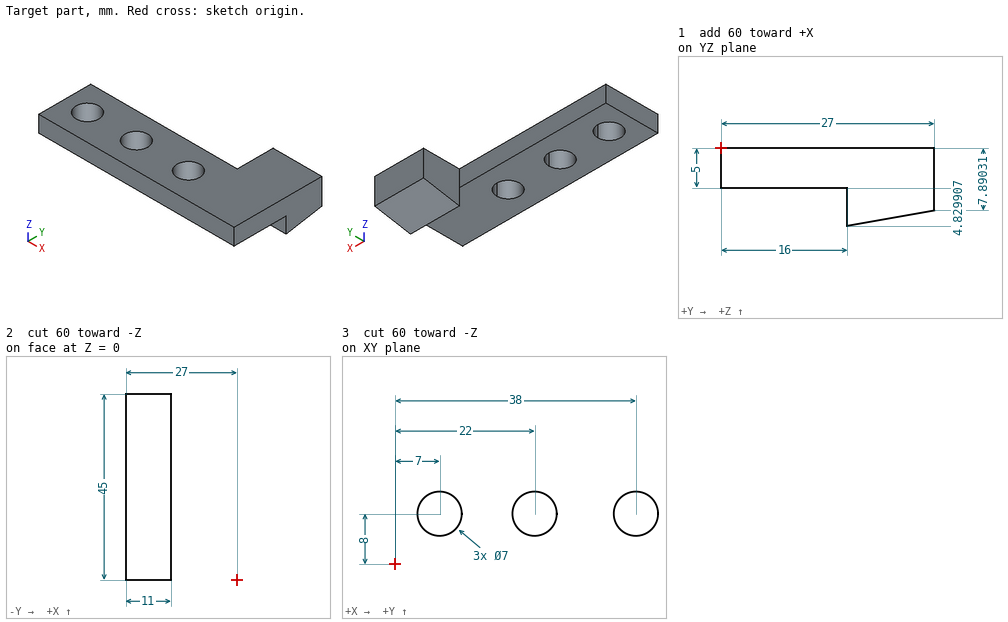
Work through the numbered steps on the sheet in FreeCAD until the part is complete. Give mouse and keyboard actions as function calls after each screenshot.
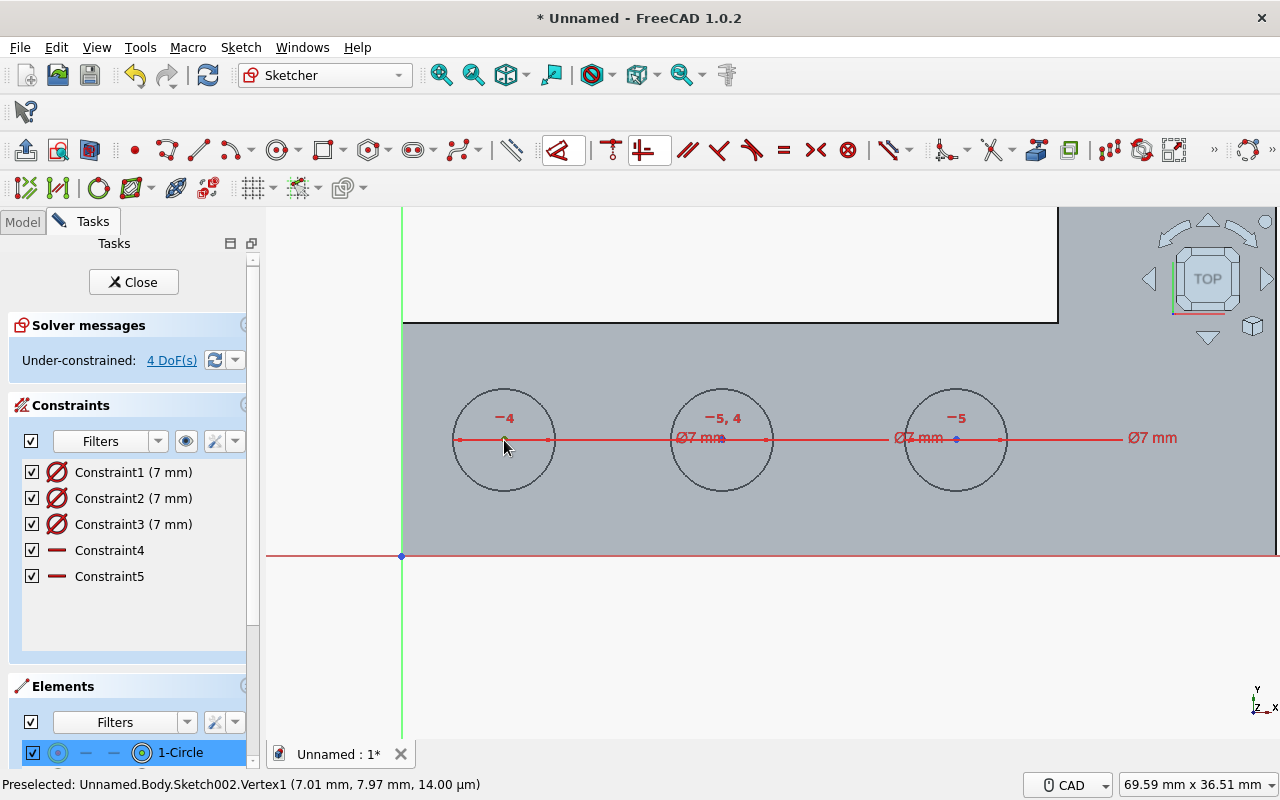
click(580, 150)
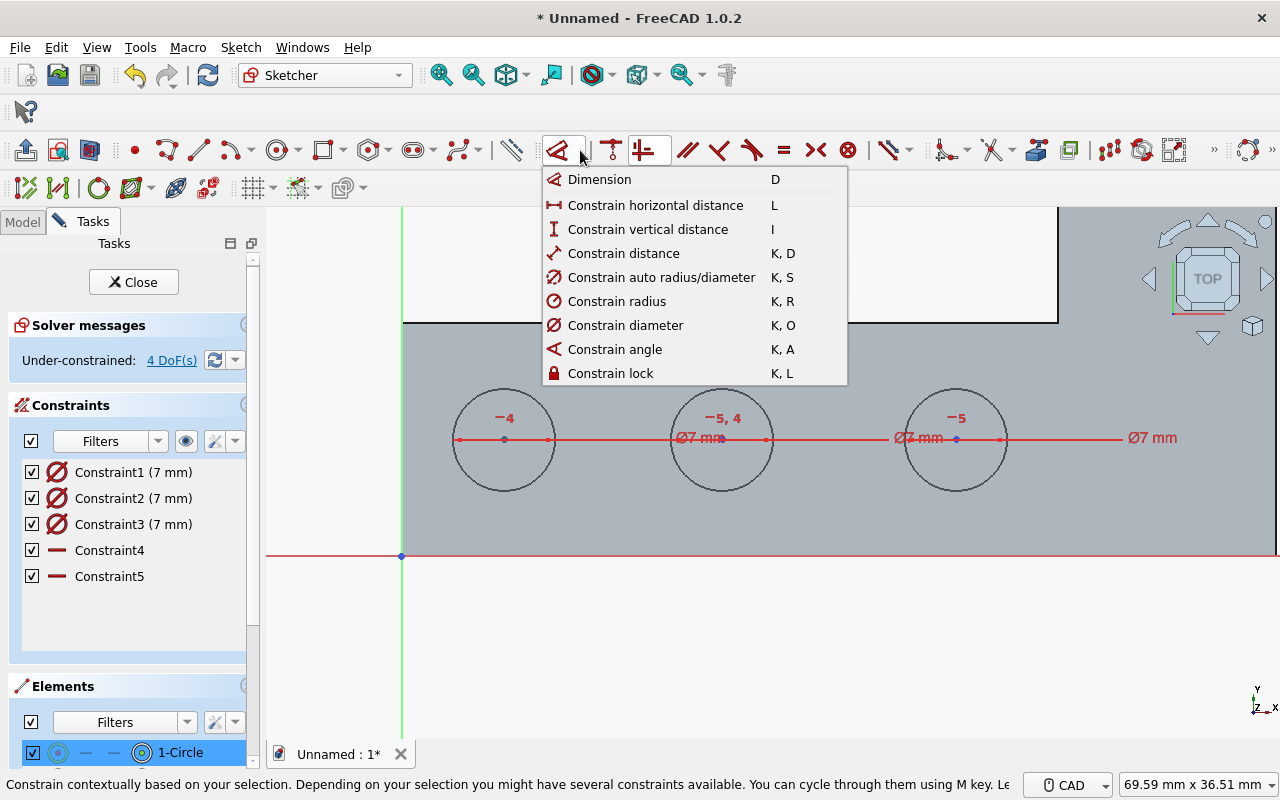
click(695, 205)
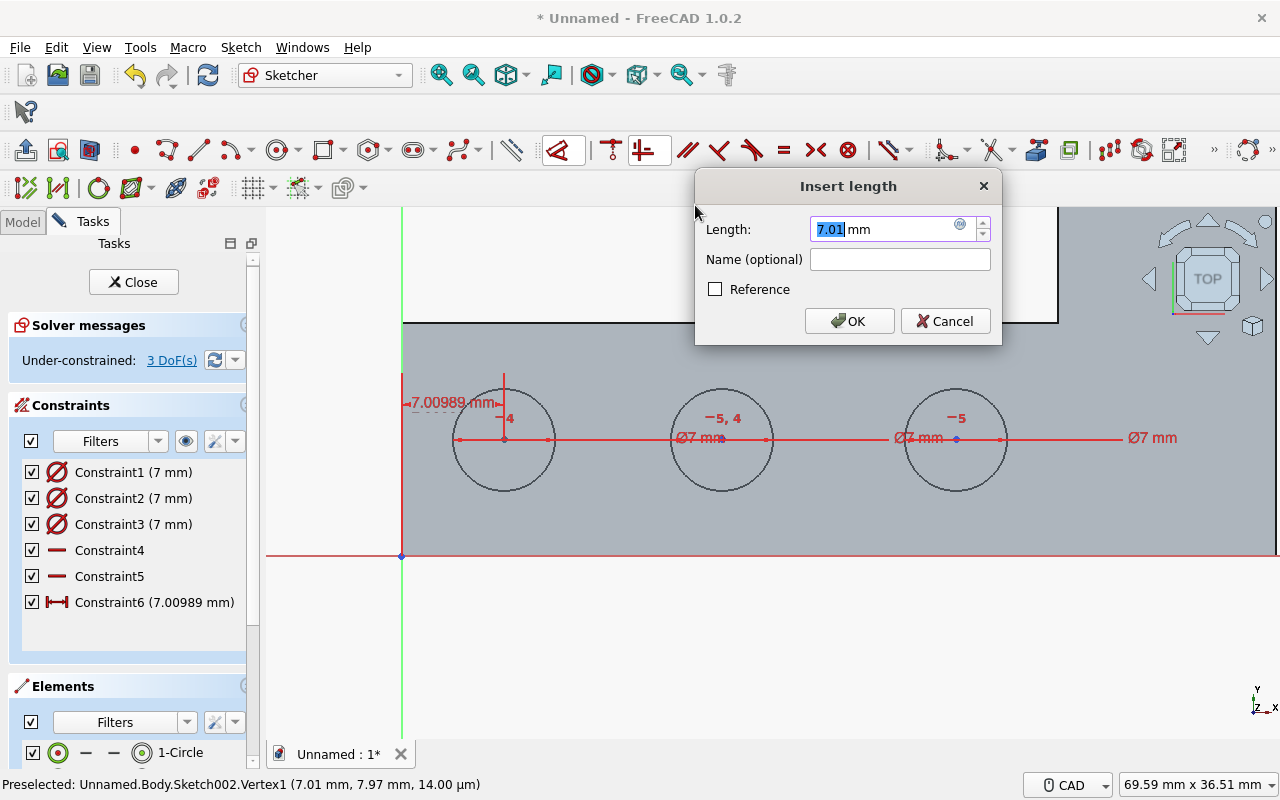
text(7)
key(Return)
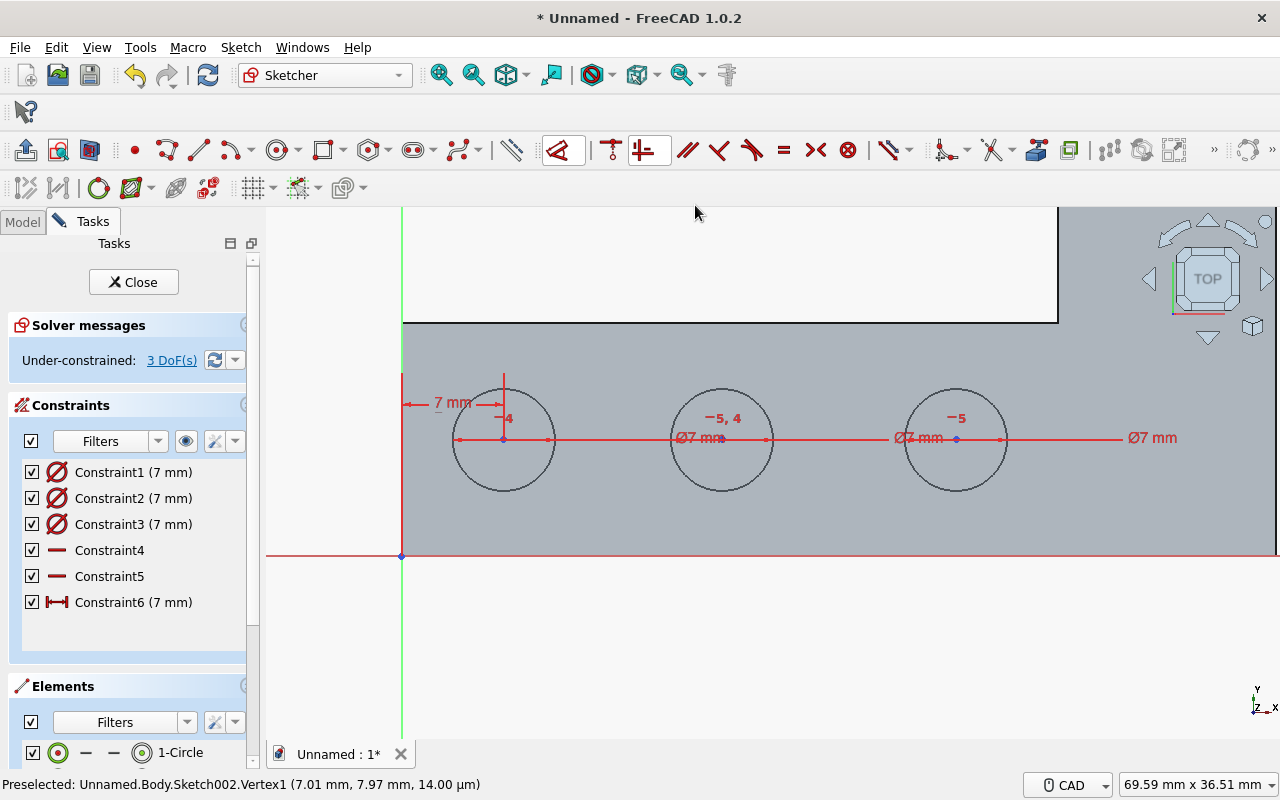
click(504, 440)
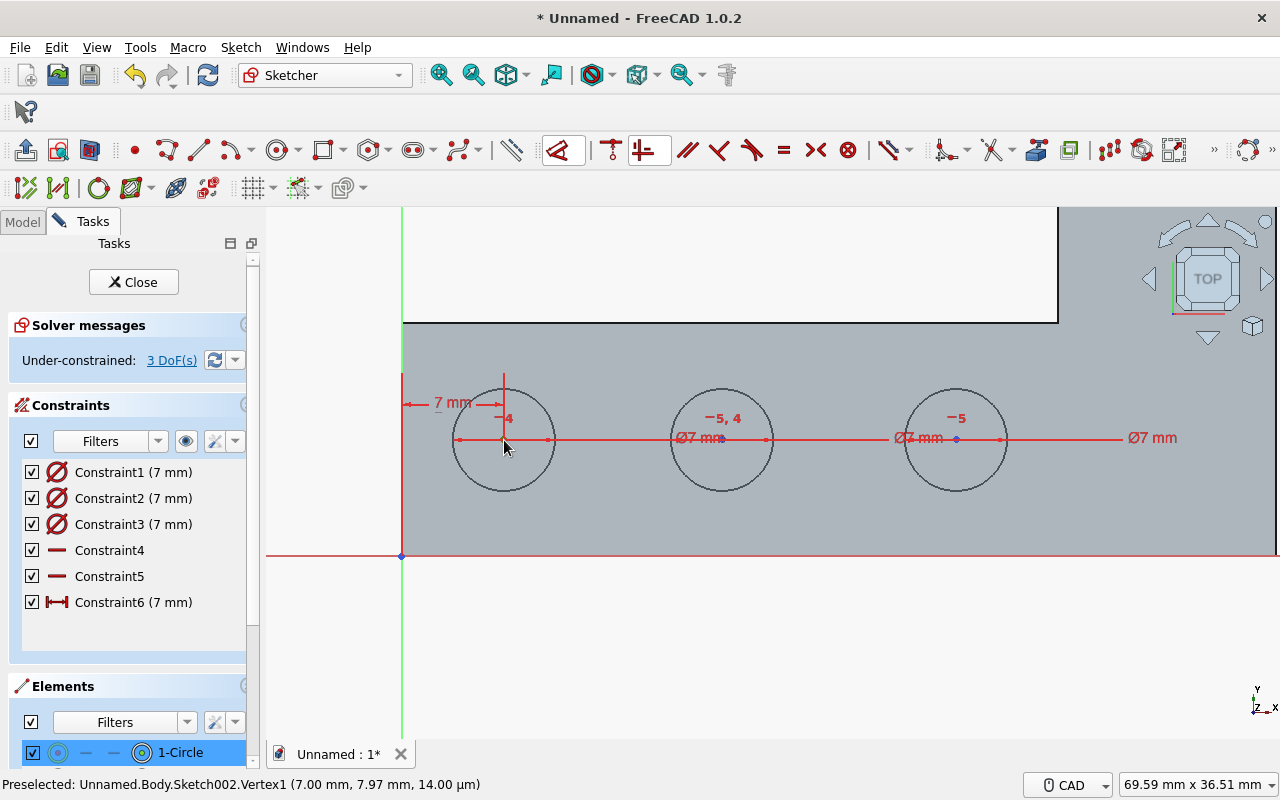
key(i)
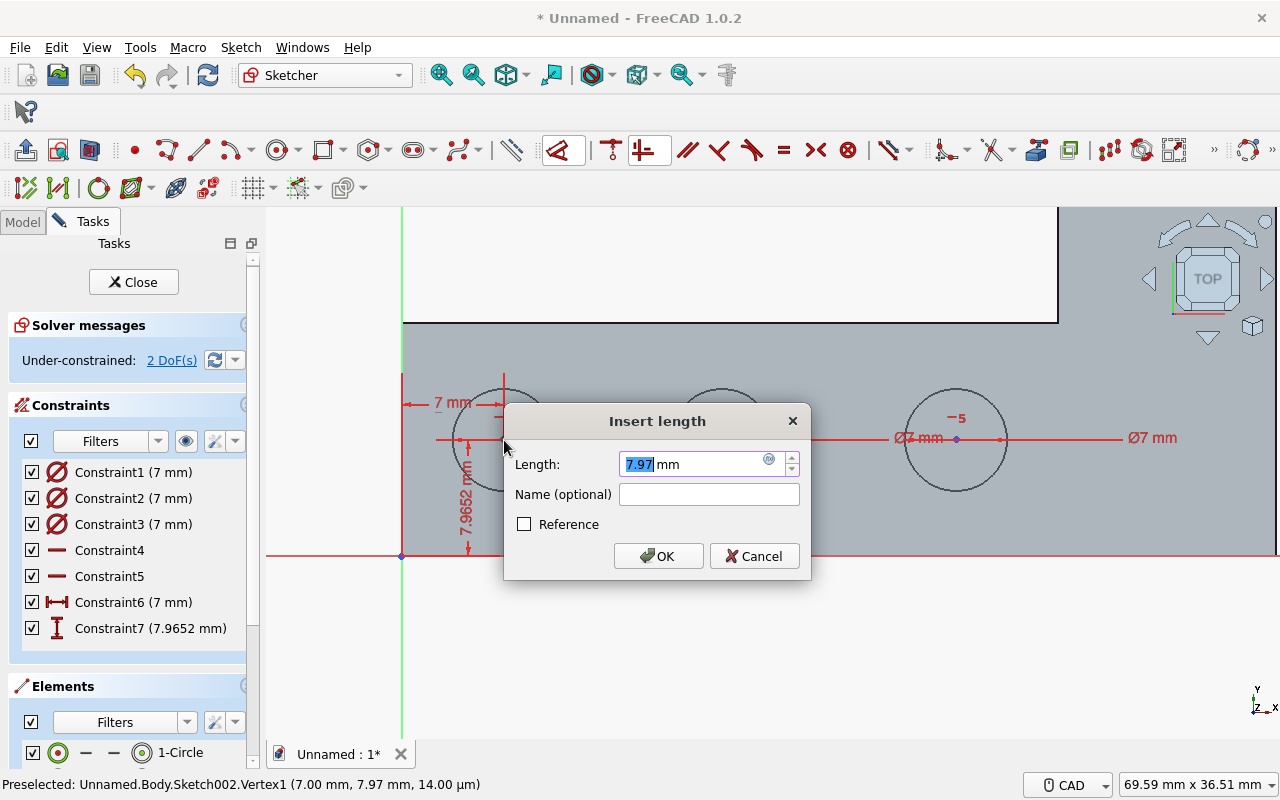
text(8)
key(Return)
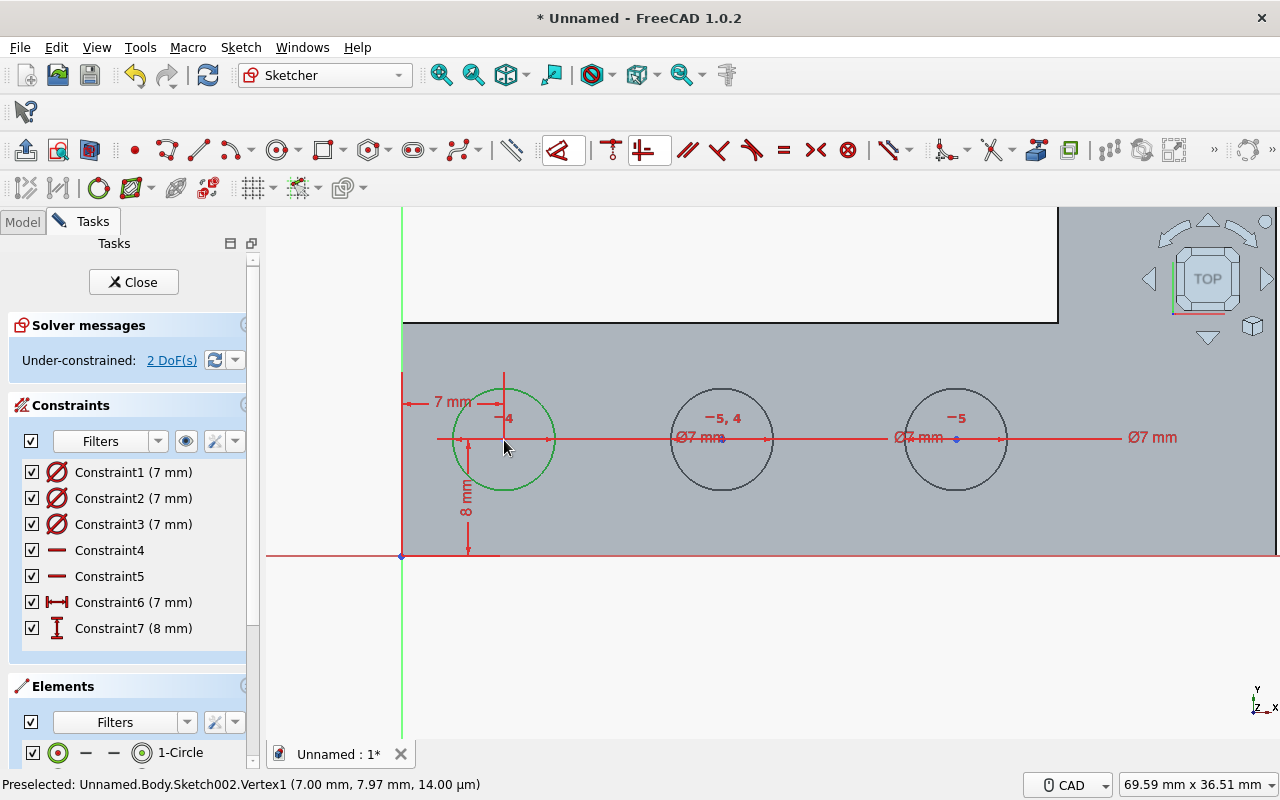
click(722, 439)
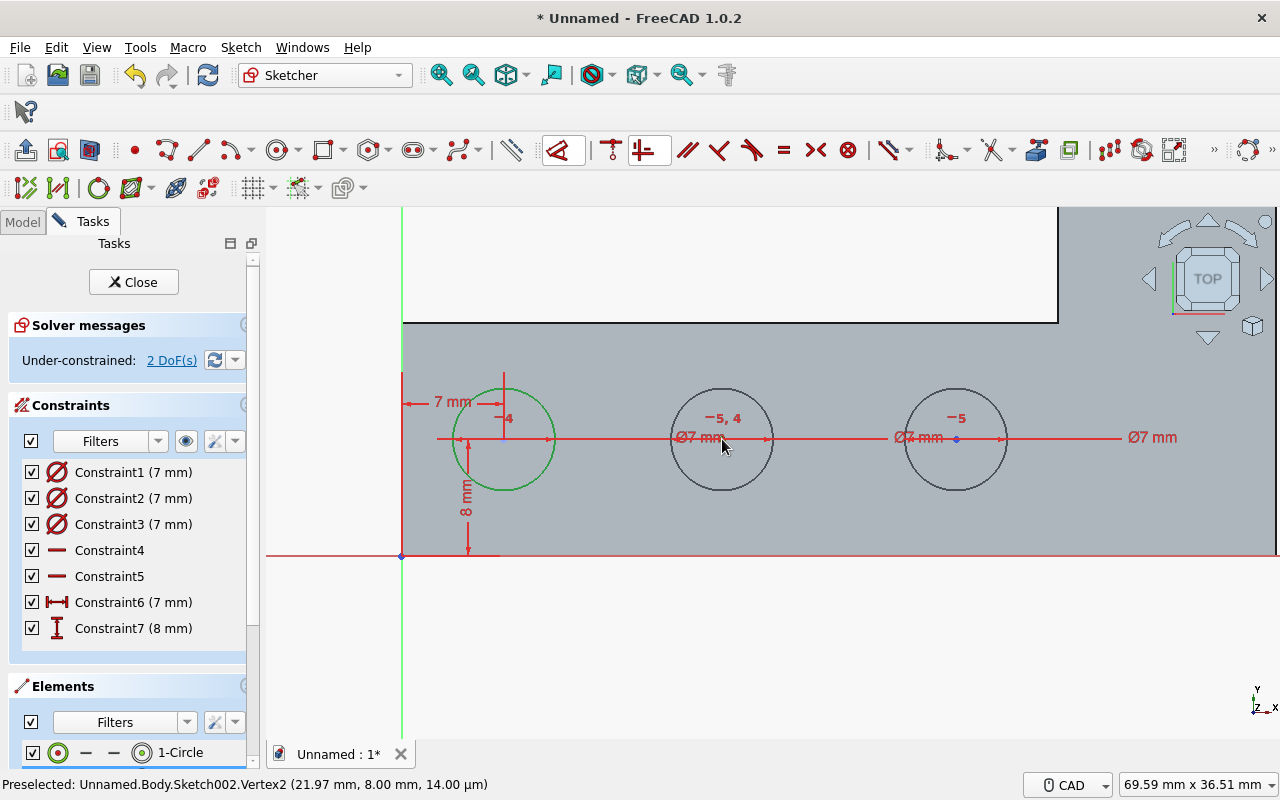
click(580, 150)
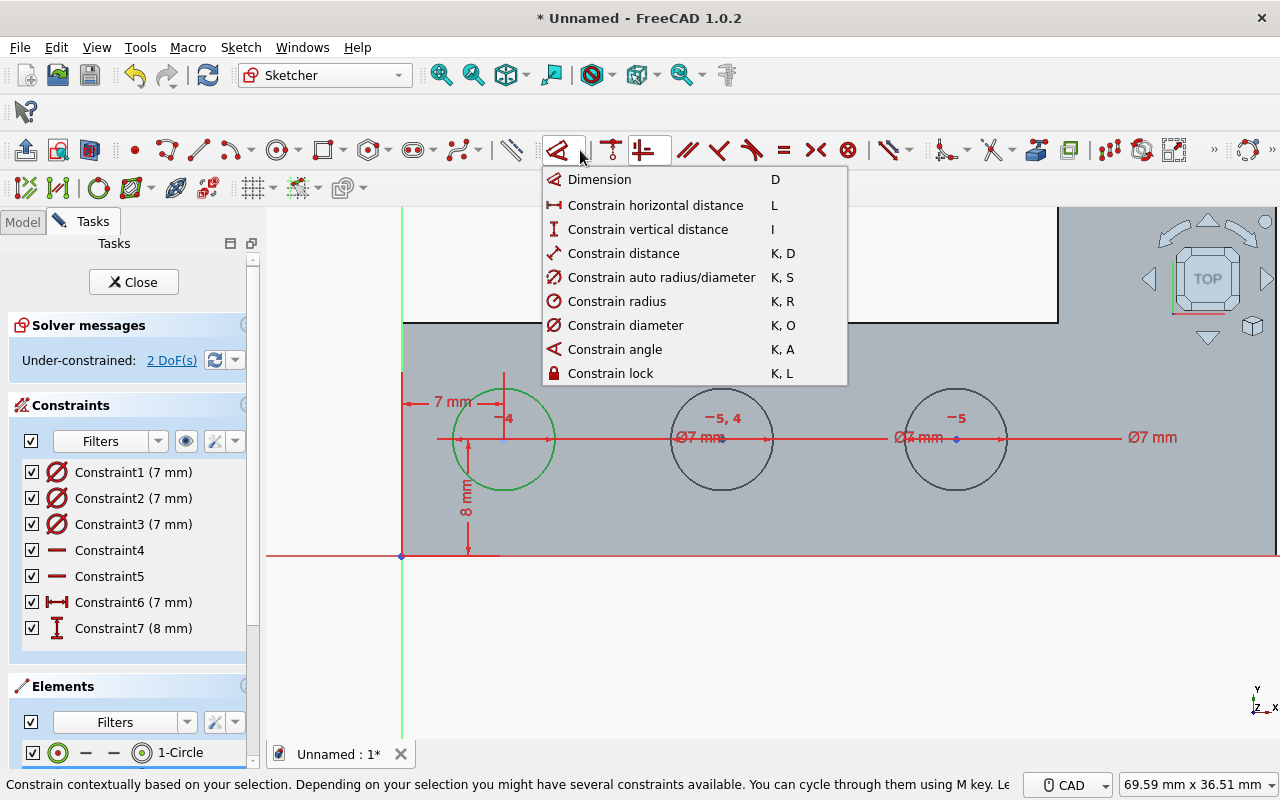
click(695, 205)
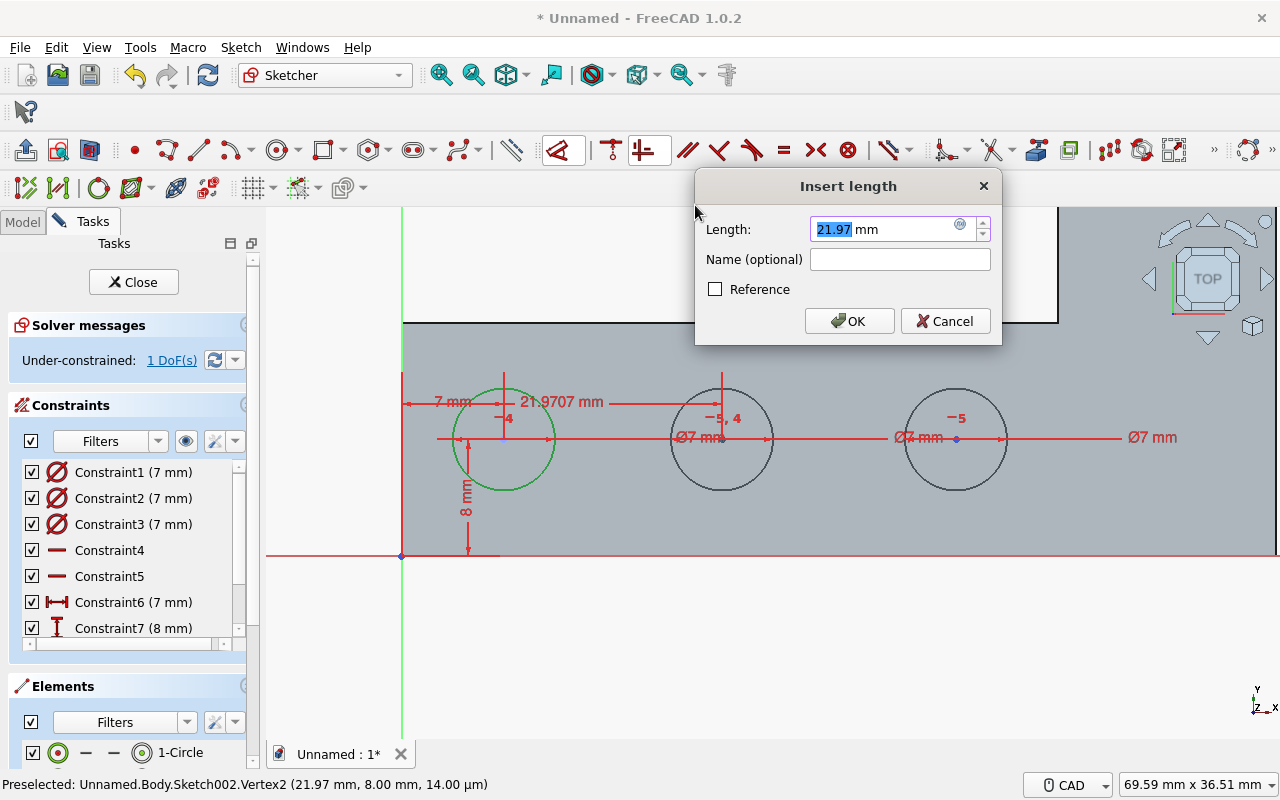
text(22)
key(Return)